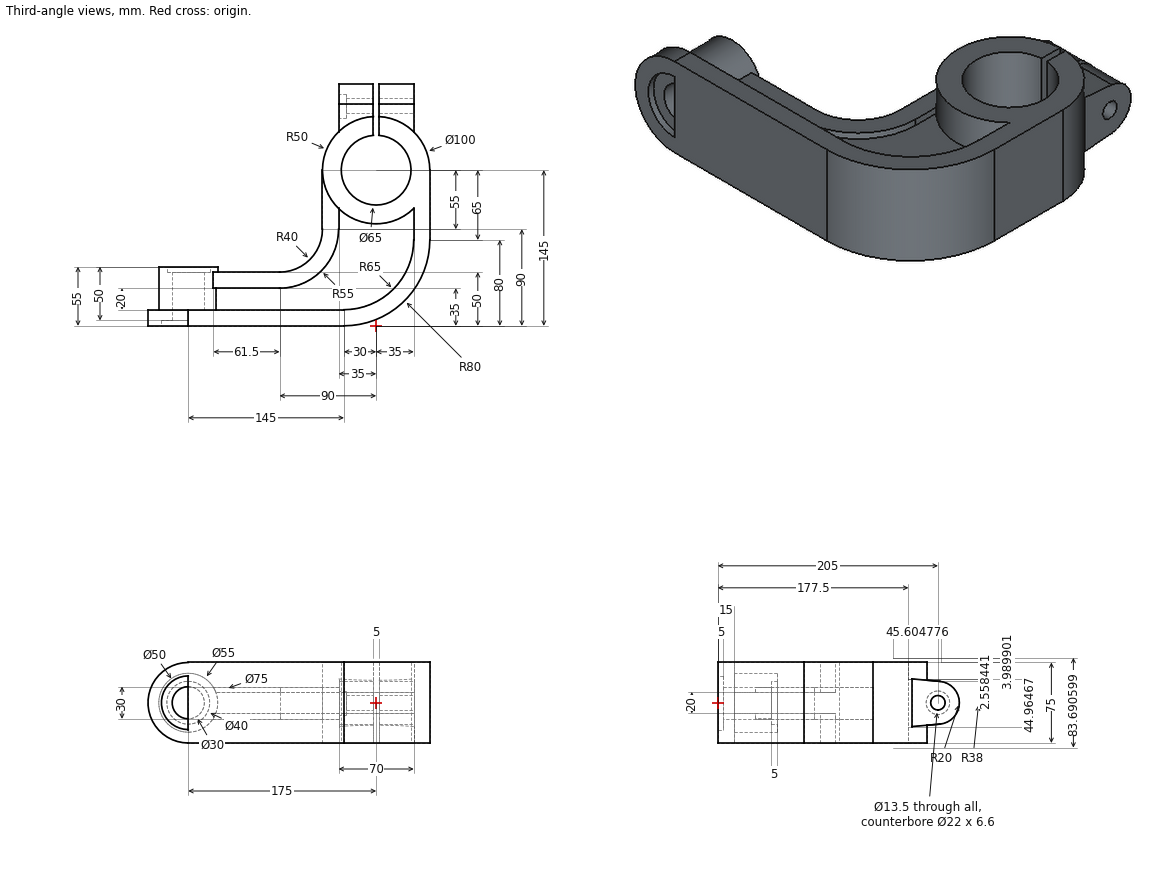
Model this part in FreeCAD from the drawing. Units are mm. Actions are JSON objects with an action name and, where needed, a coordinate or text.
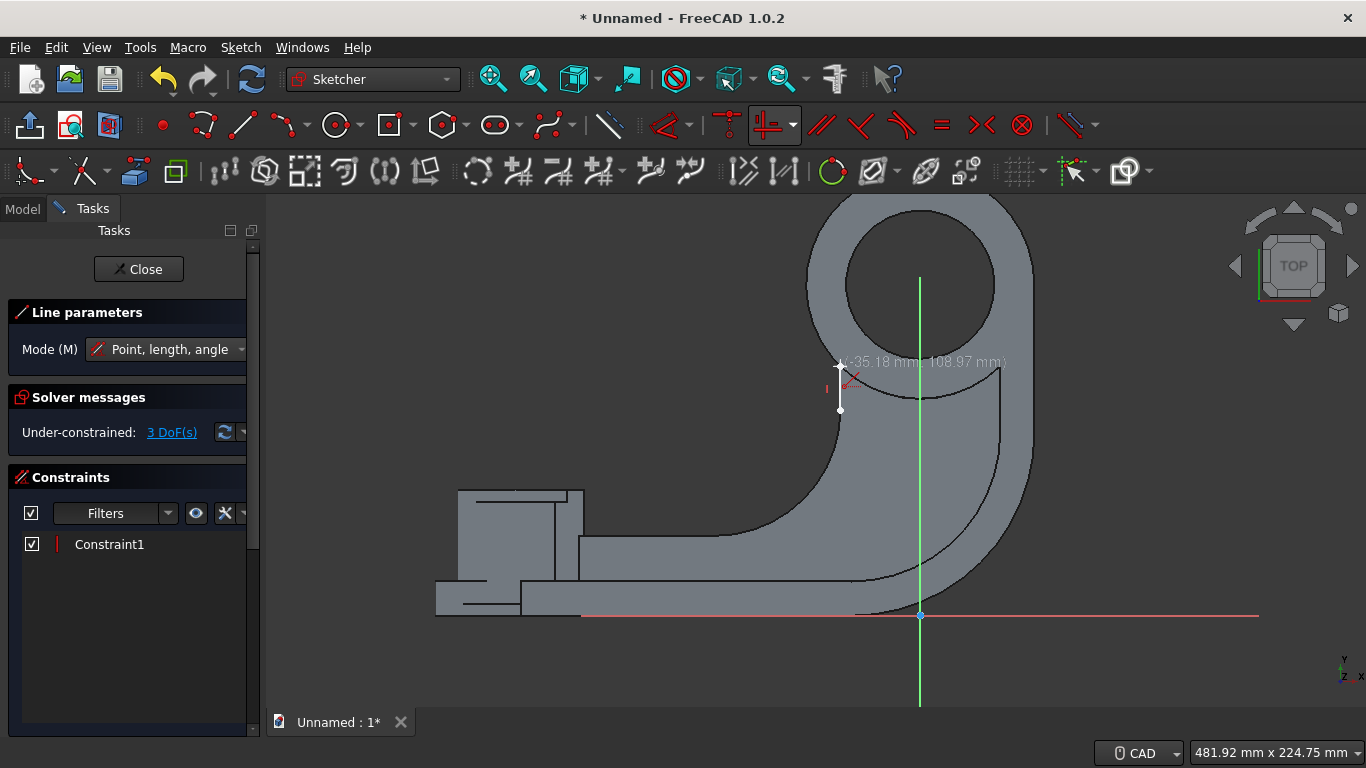
{"action": "left_click", "coordinate": [806, 285]}
{"action": "left_click", "coordinate": [806, 410]}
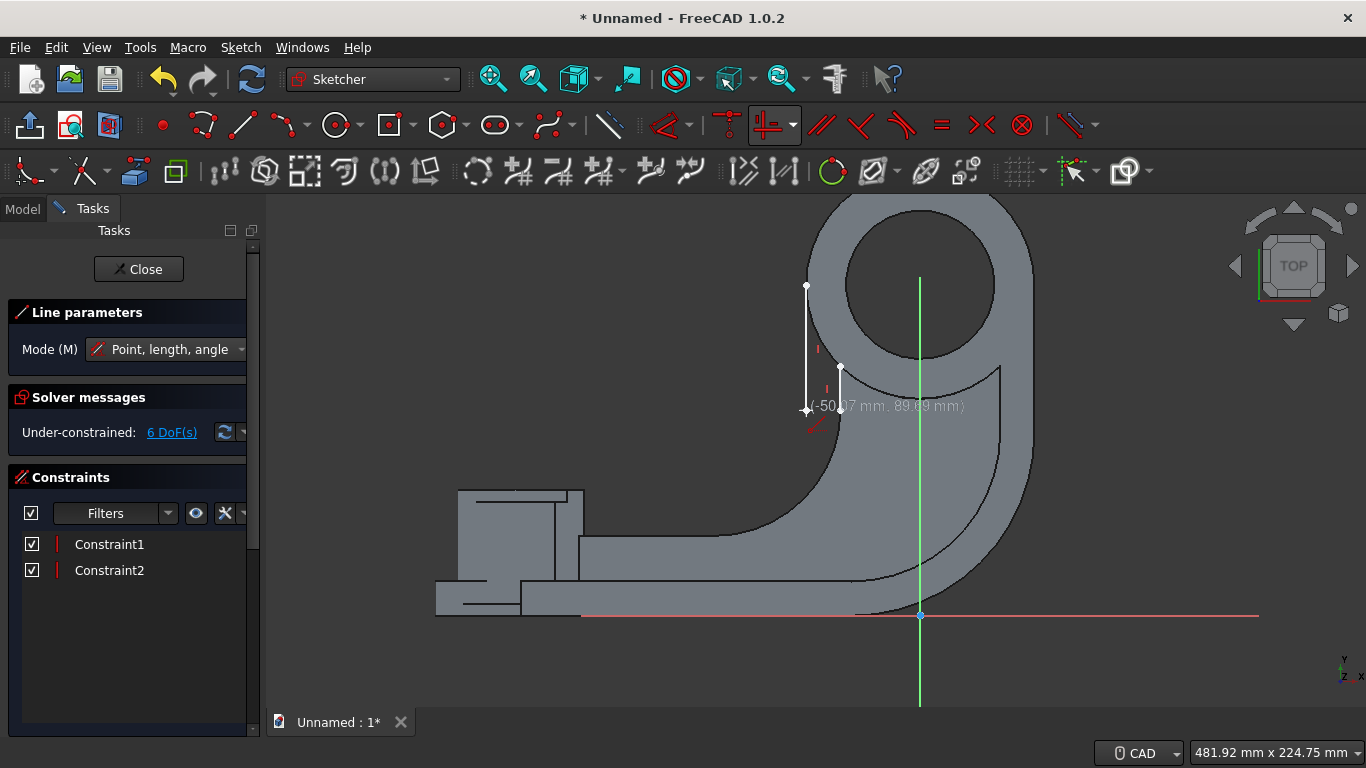
{"action": "left_click", "coordinate": [204, 126]}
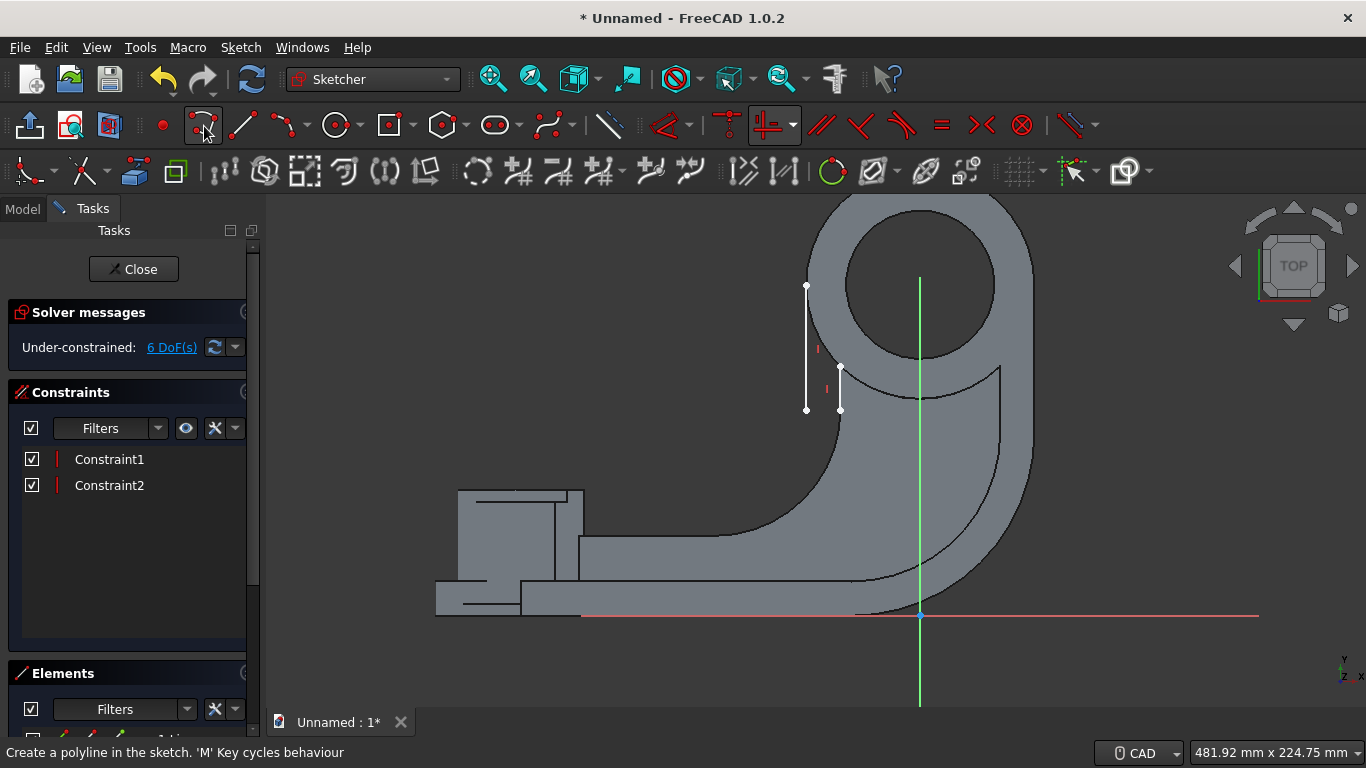
{"action": "left_click", "coordinate": [715, 502]}
{"action": "left_click", "coordinate": [574, 502]}
{"action": "left_click", "coordinate": [574, 536]}
{"action": "left_click", "coordinate": [715, 536]}
{"action": "right_click", "coordinate": [715, 536]}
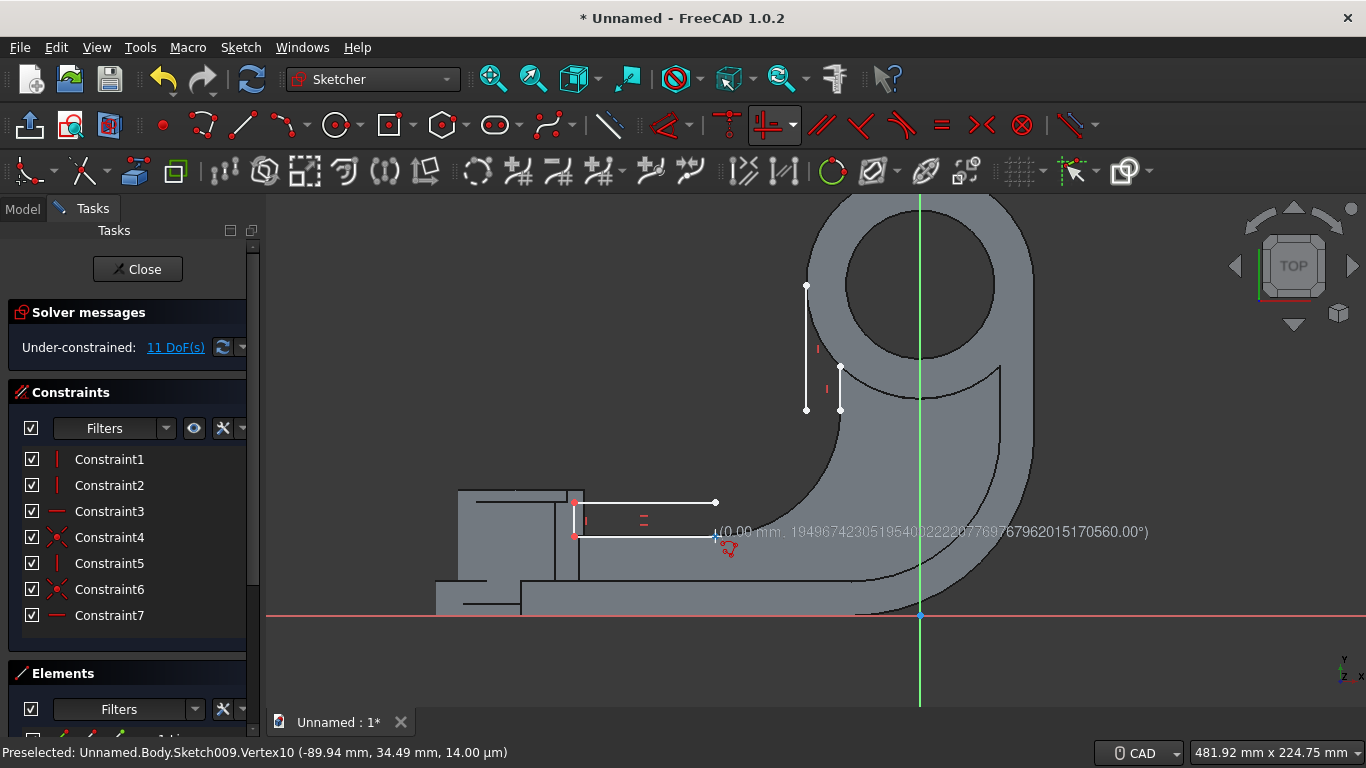
{"action": "key", "text": "g 3 a"}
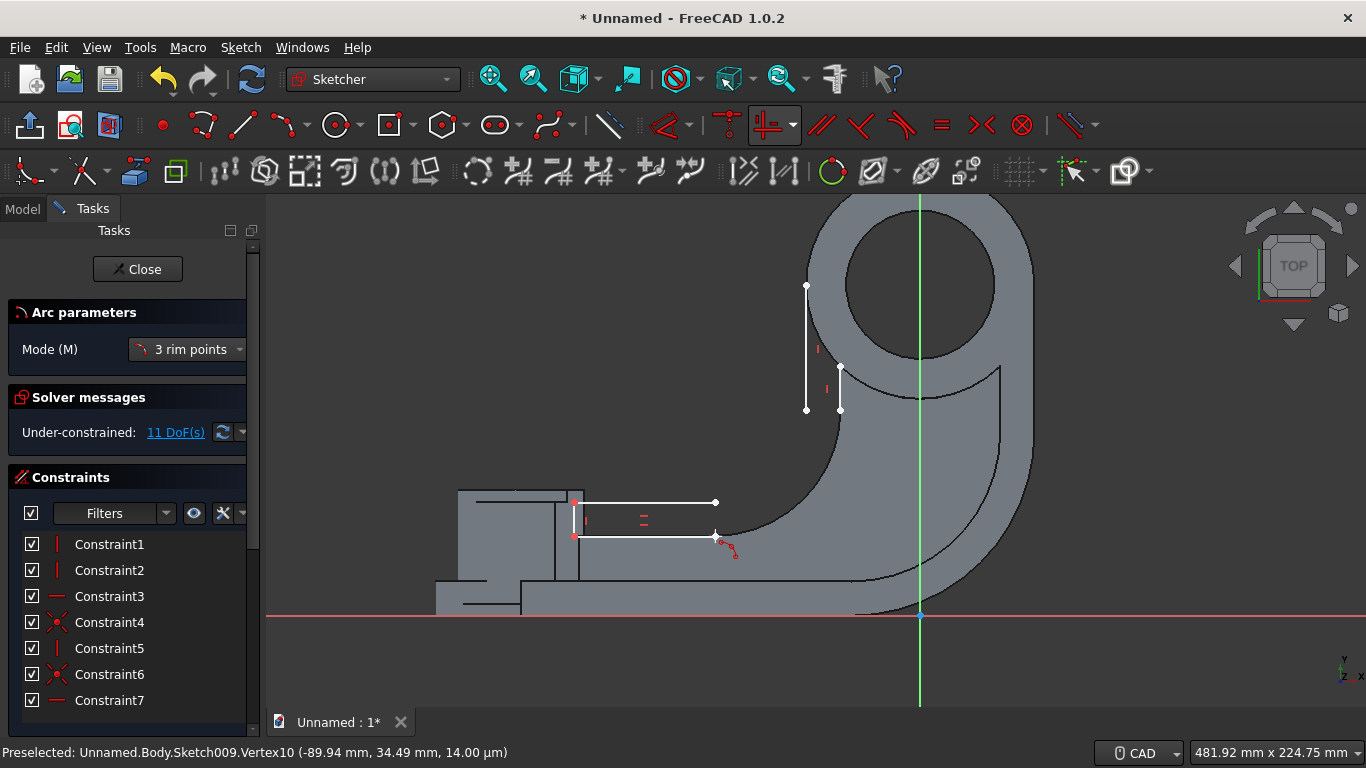
{"action": "left_click", "coordinate": [840, 367]}
{"action": "left_click", "coordinate": [806, 286]}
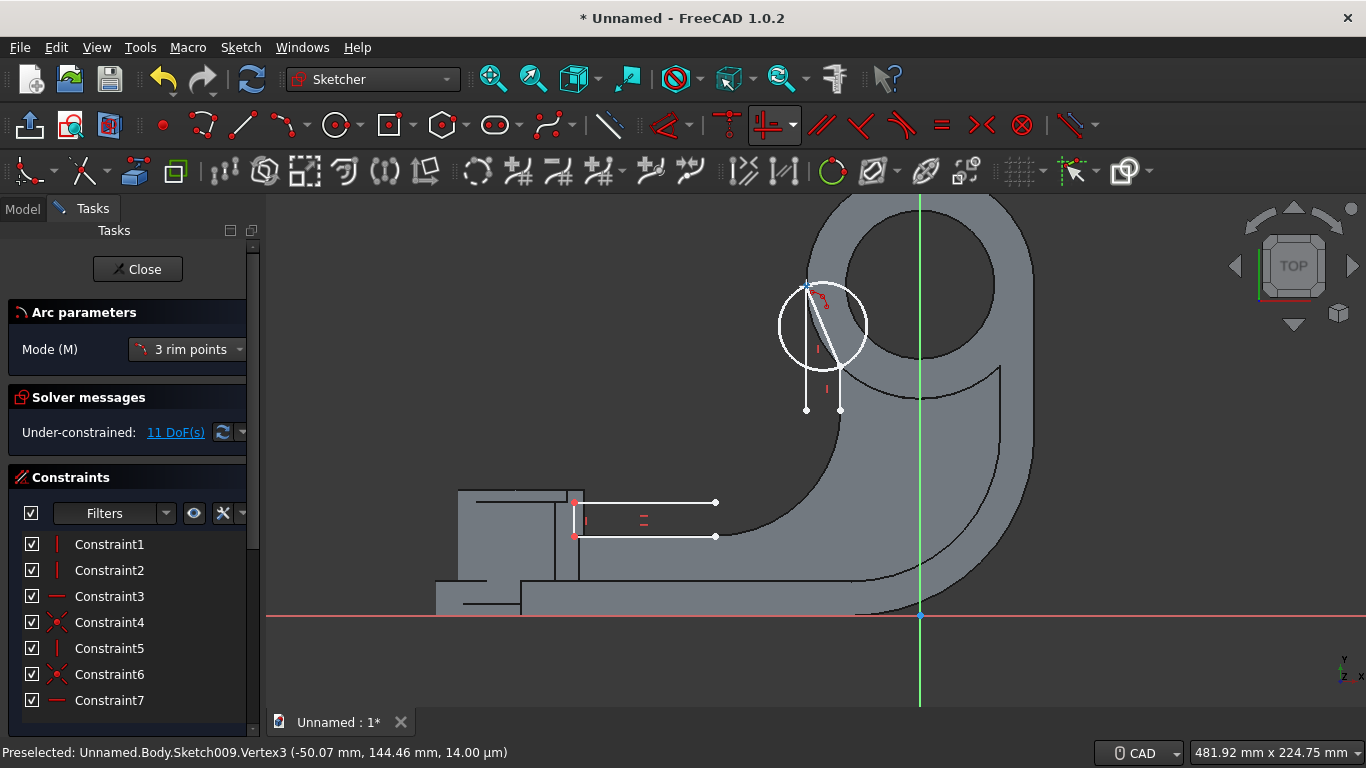
{"action": "scroll", "coordinate": [815, 329], "scroll_direction": "up", "scroll_amount": 3}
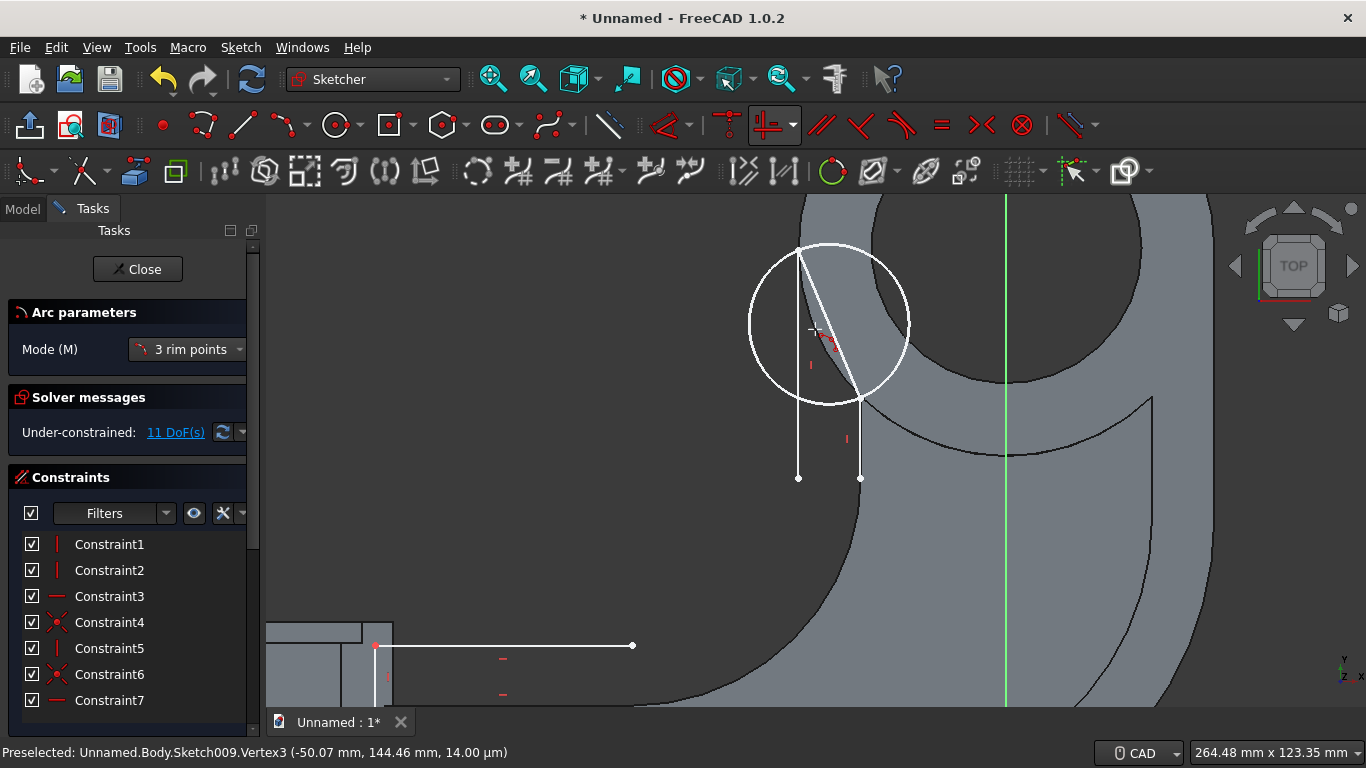
{"action": "left_click", "coordinate": [815, 329]}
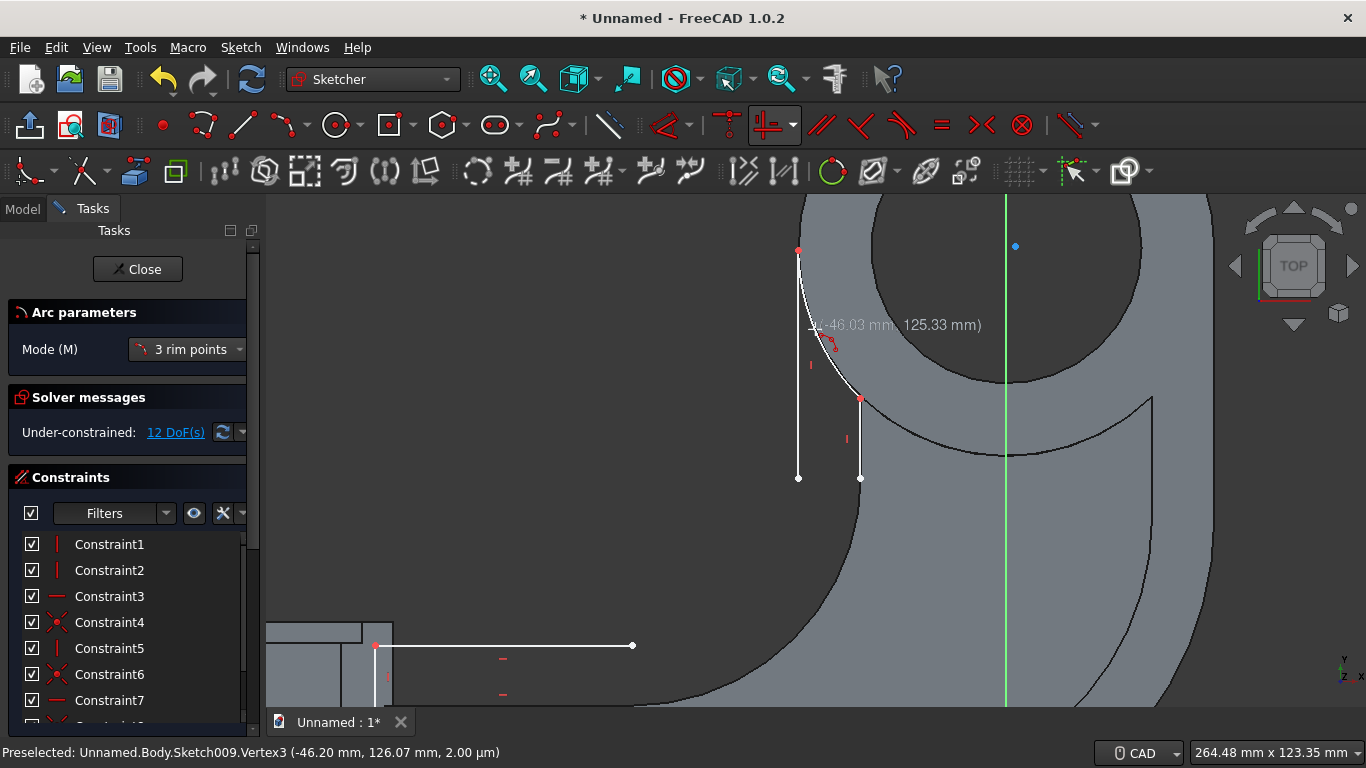
{"action": "left_click", "coordinate": [798, 478]}
{"action": "left_click", "coordinate": [632, 646]}
{"action": "left_click", "coordinate": [750, 595]}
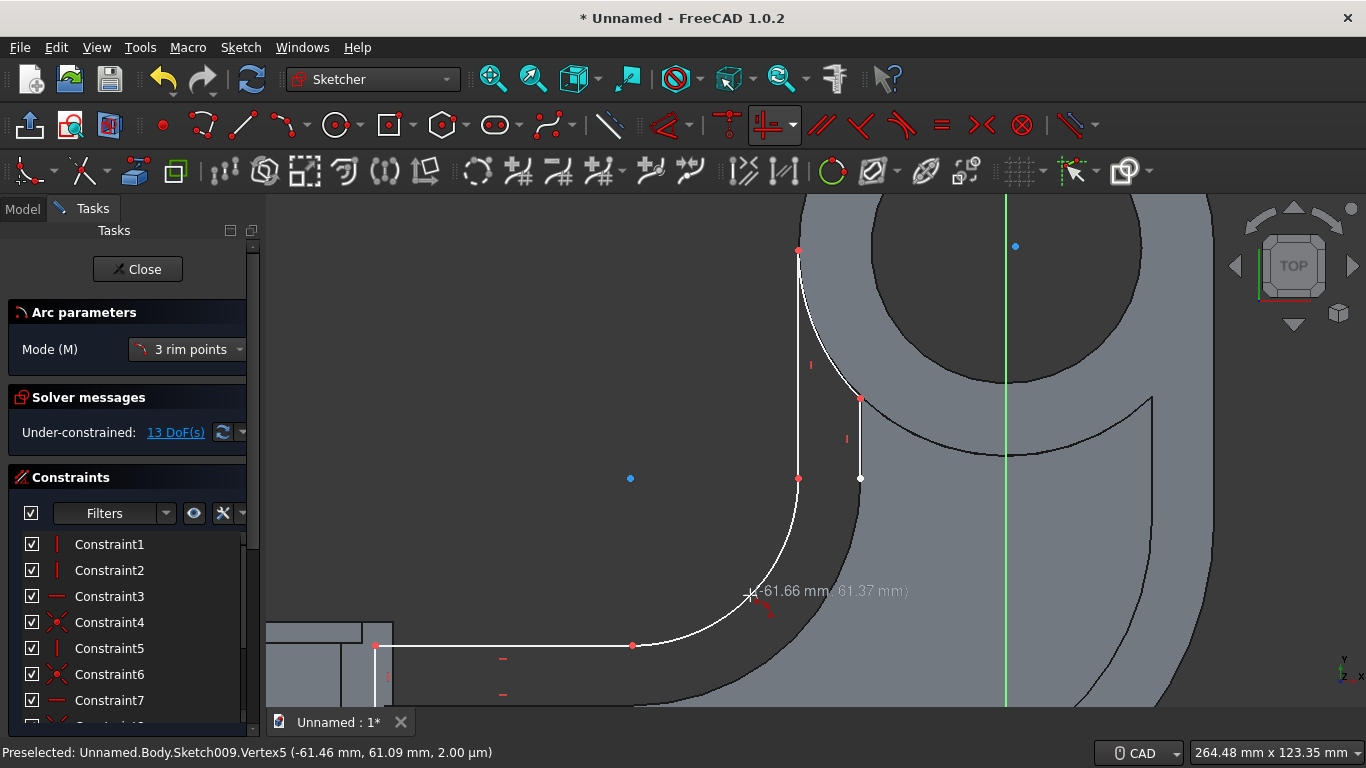
{"action": "scroll", "coordinate": [816, 330], "scroll_direction": "down", "scroll_amount": 3}